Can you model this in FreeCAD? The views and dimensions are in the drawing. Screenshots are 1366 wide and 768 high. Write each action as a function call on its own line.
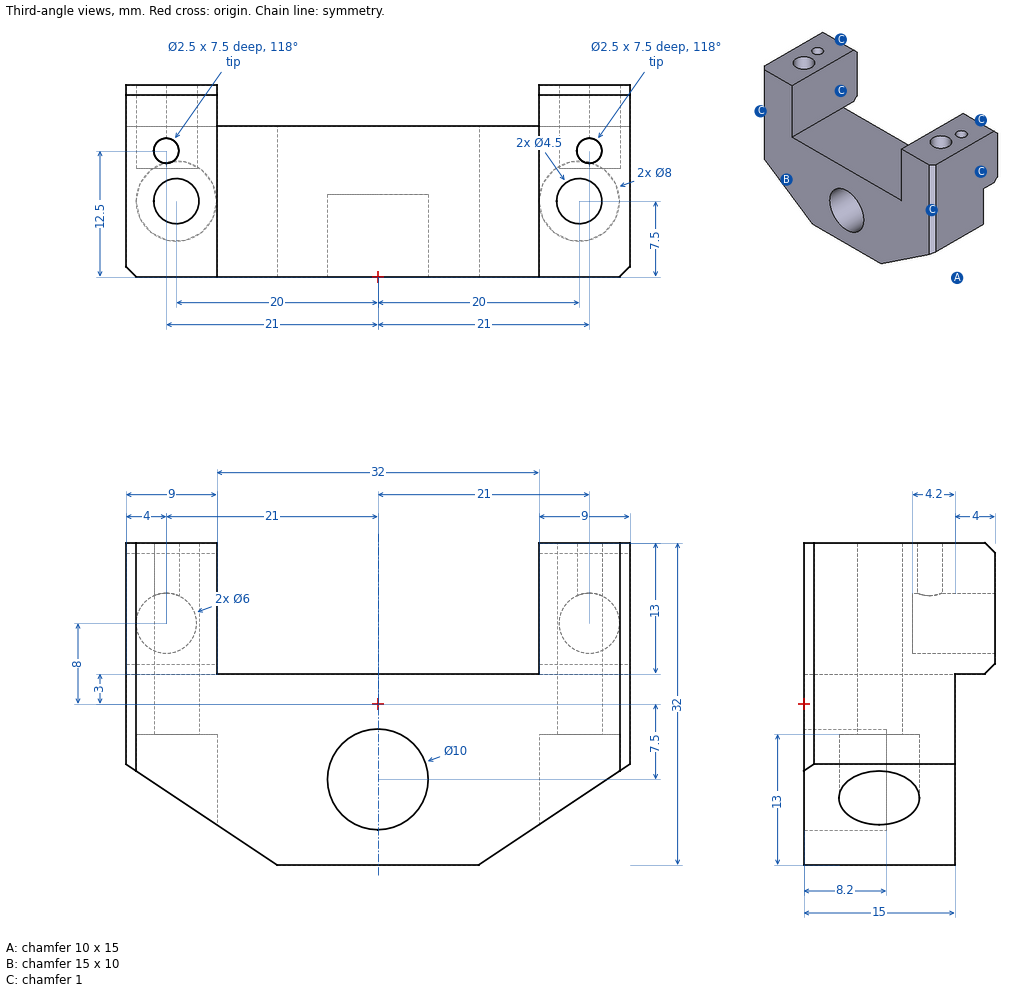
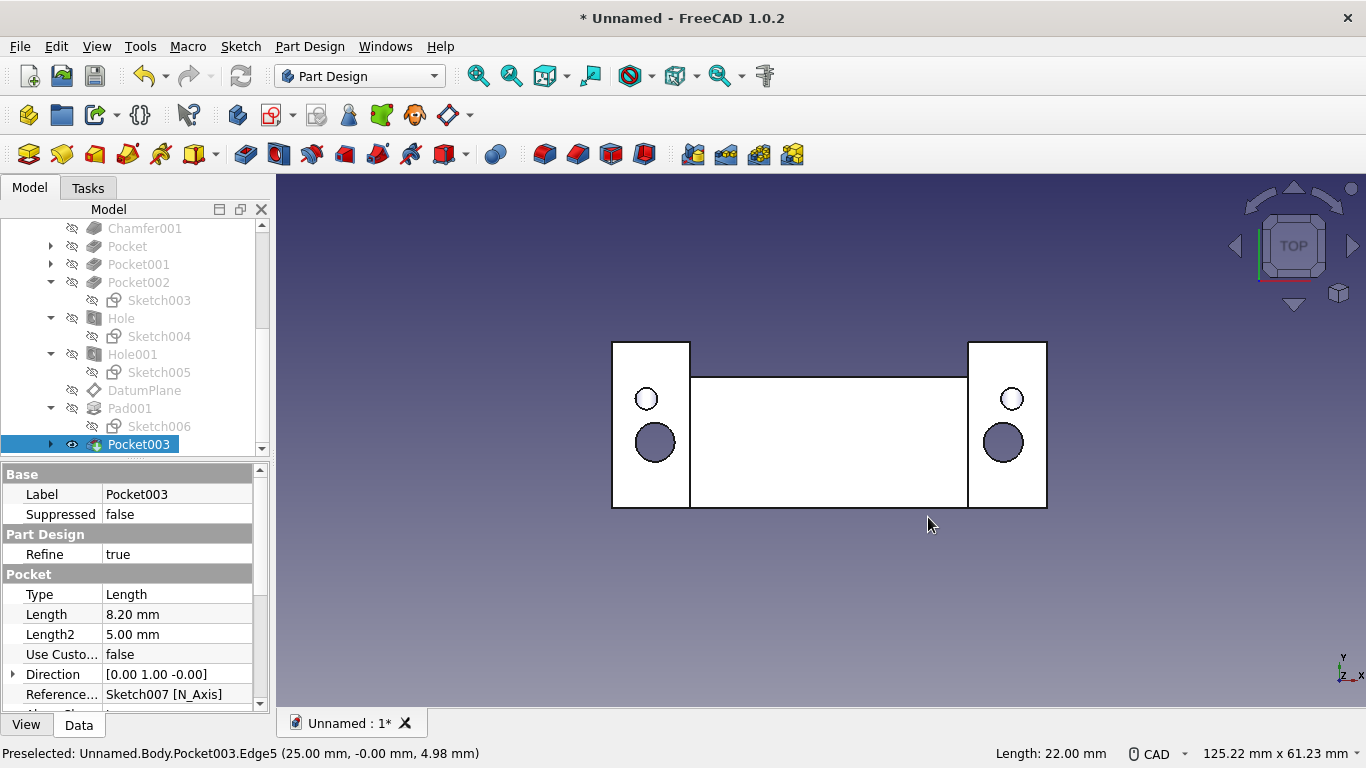
click(479, 76)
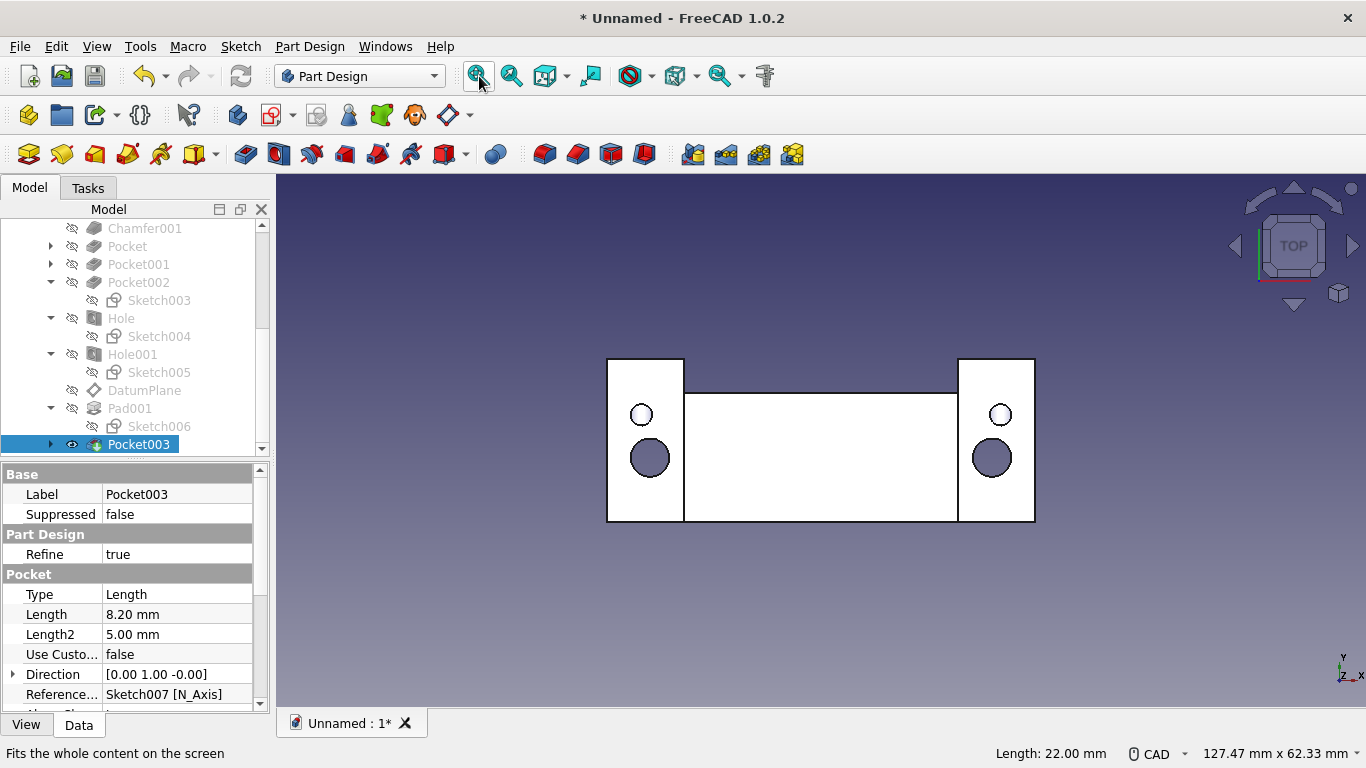
click(646, 358, ctrl)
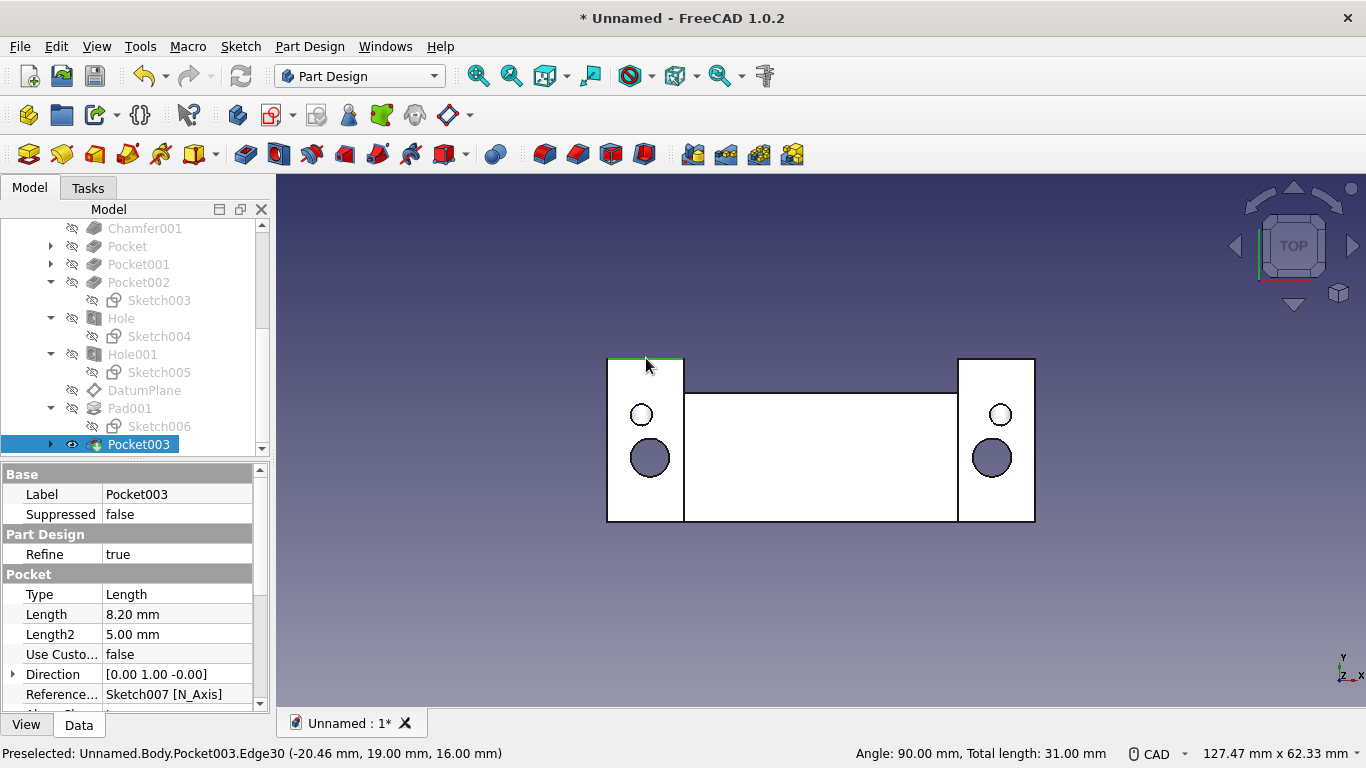
click(996, 358, ctrl)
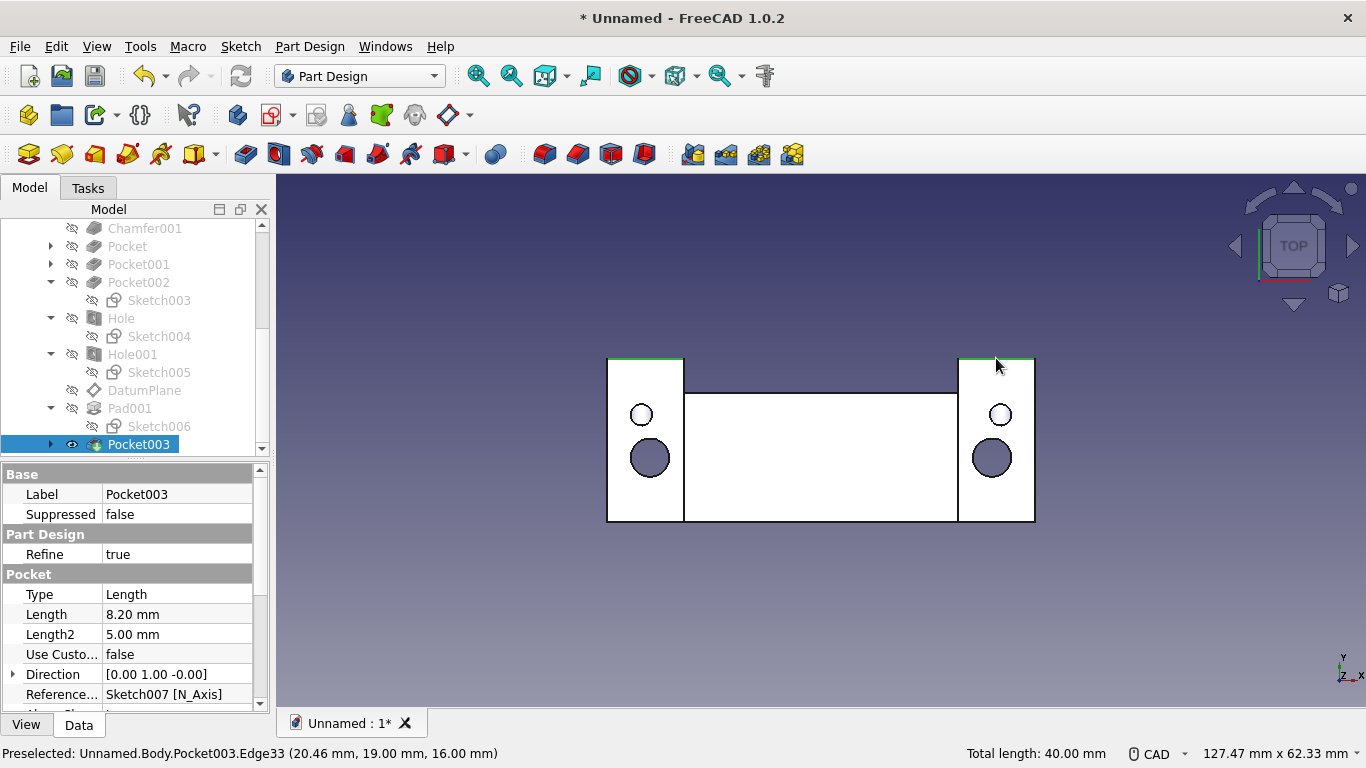
key(0)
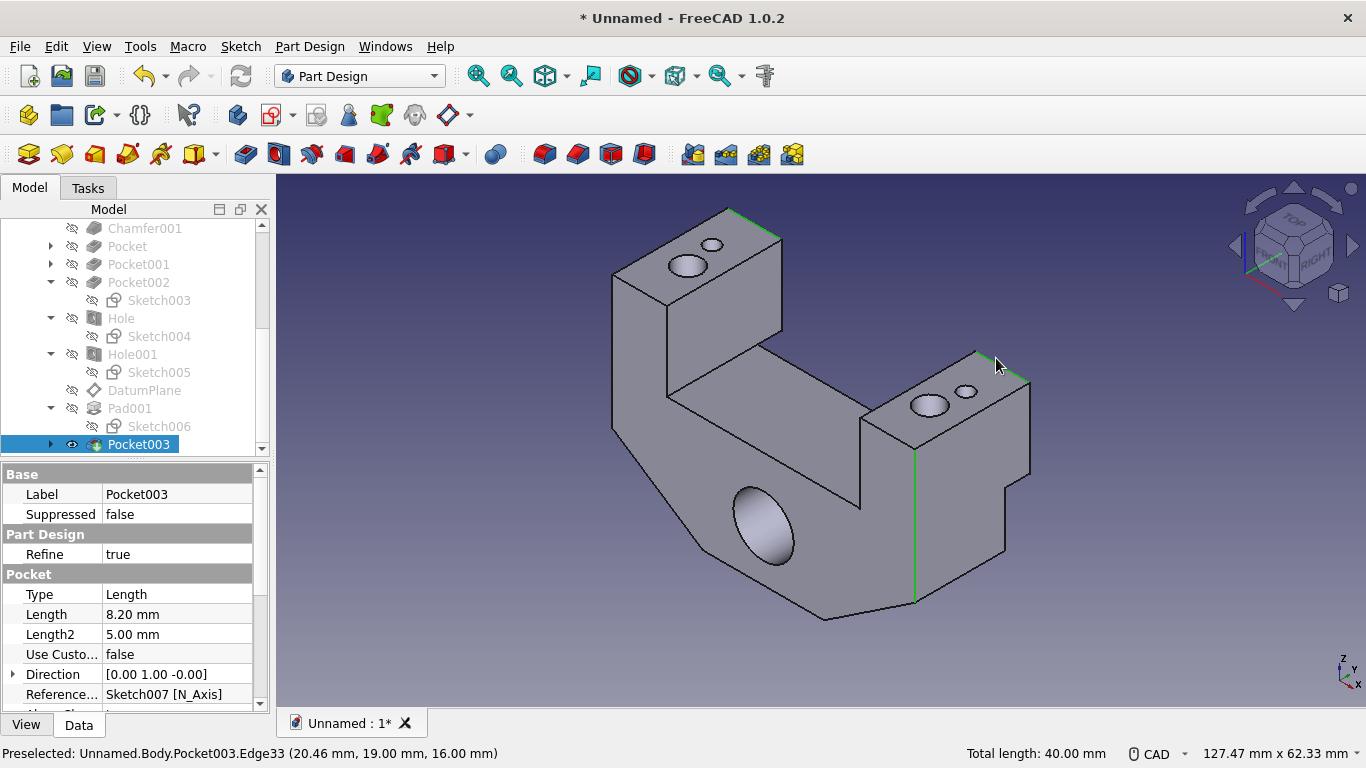
key(1)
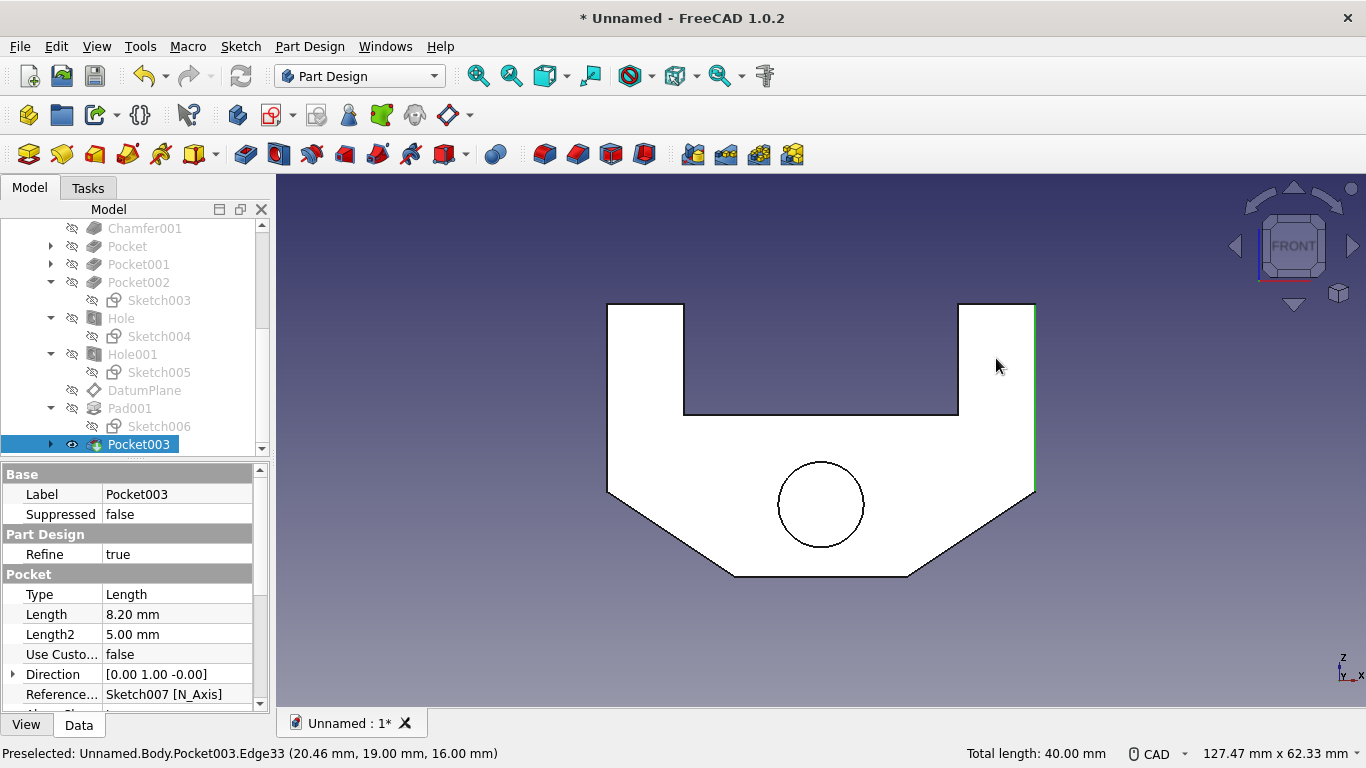
click(607, 434, ctrl)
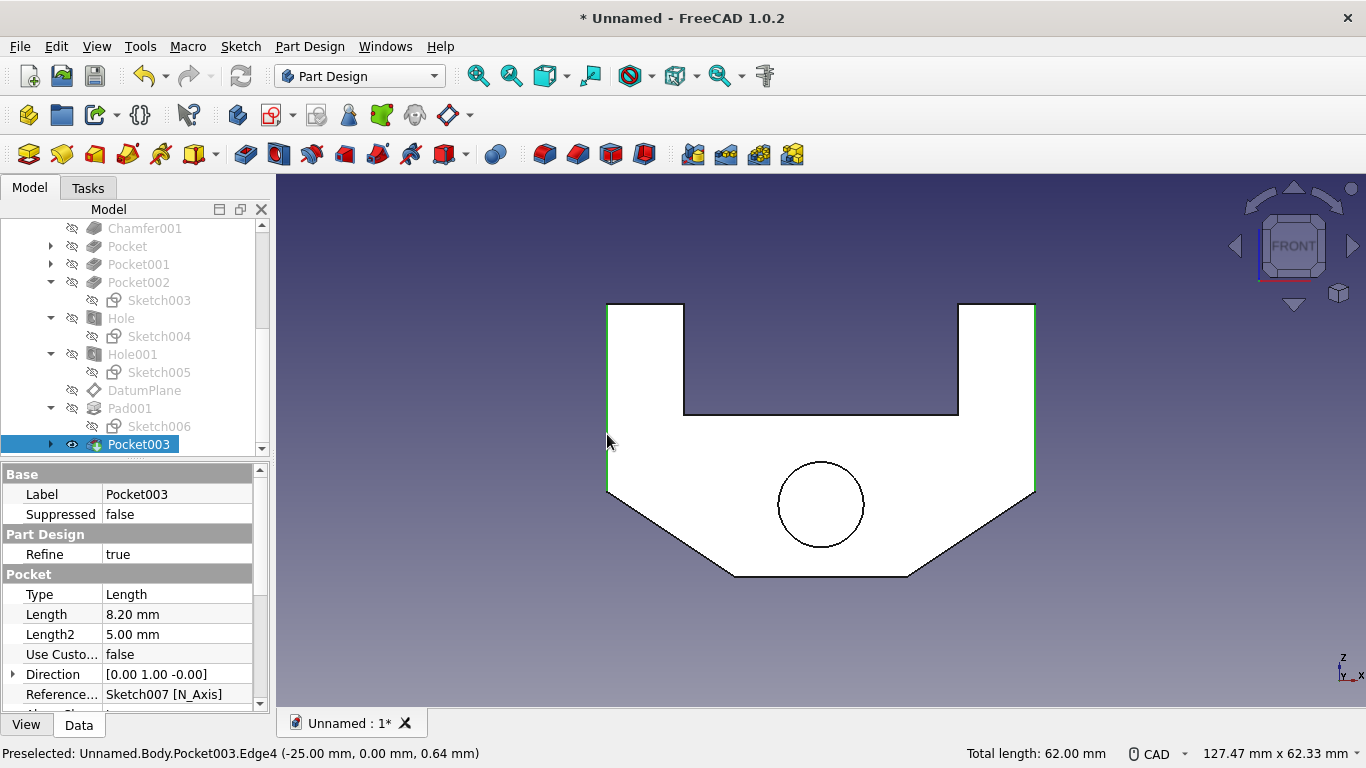
key(3)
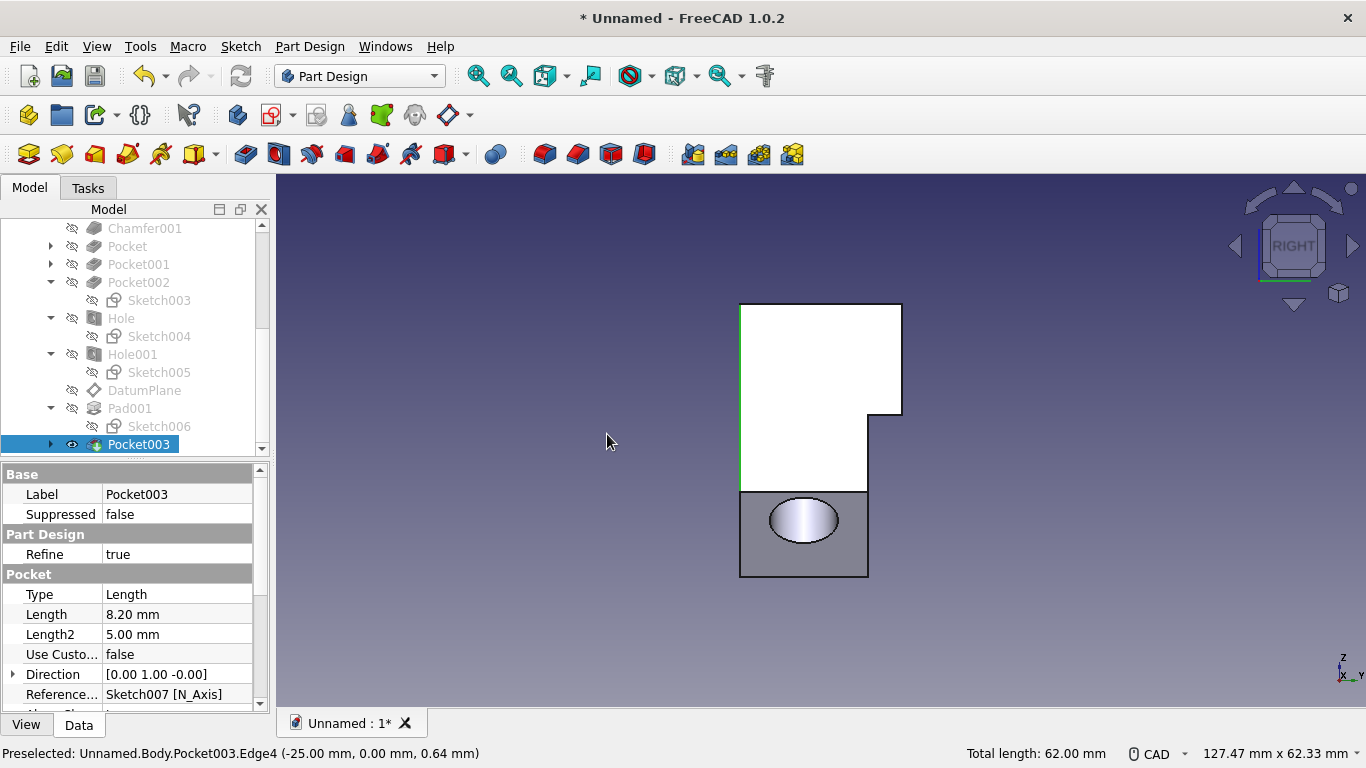
key(5)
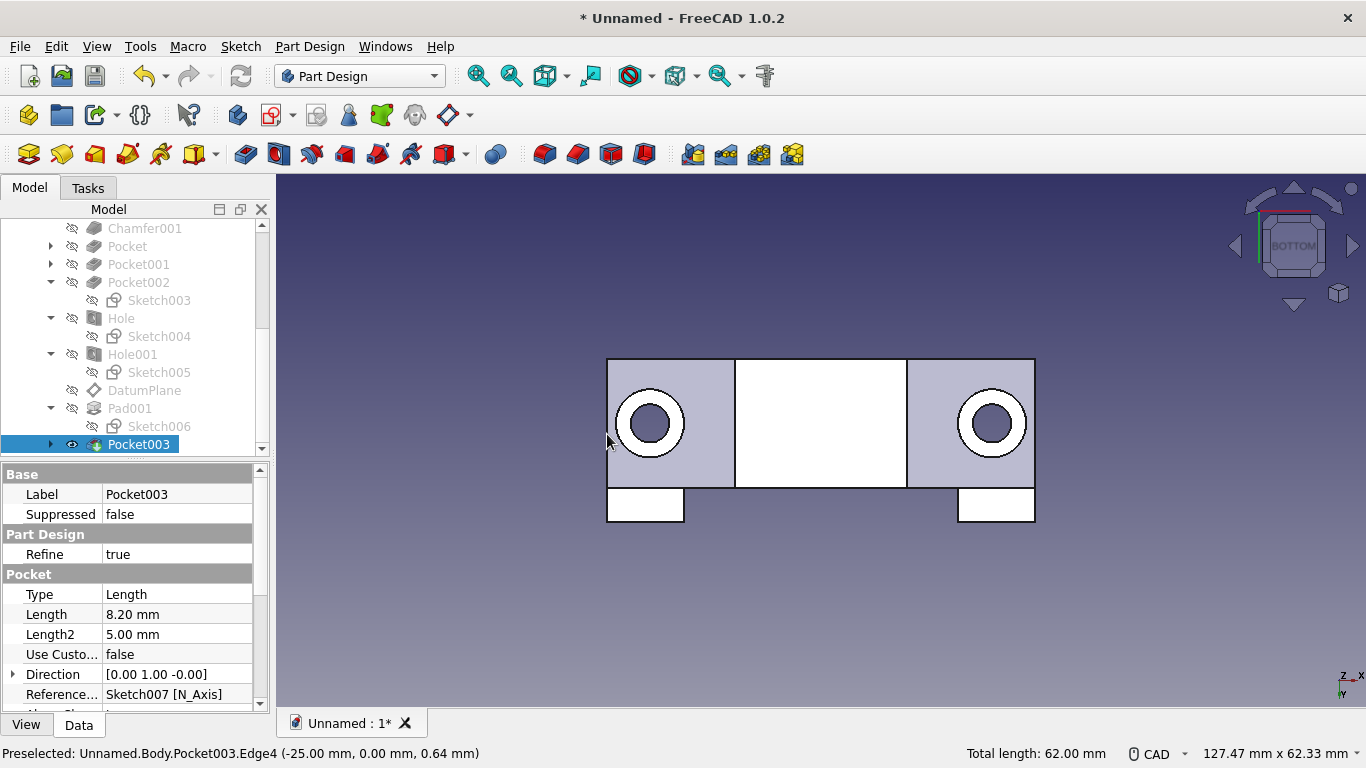
click(479, 76)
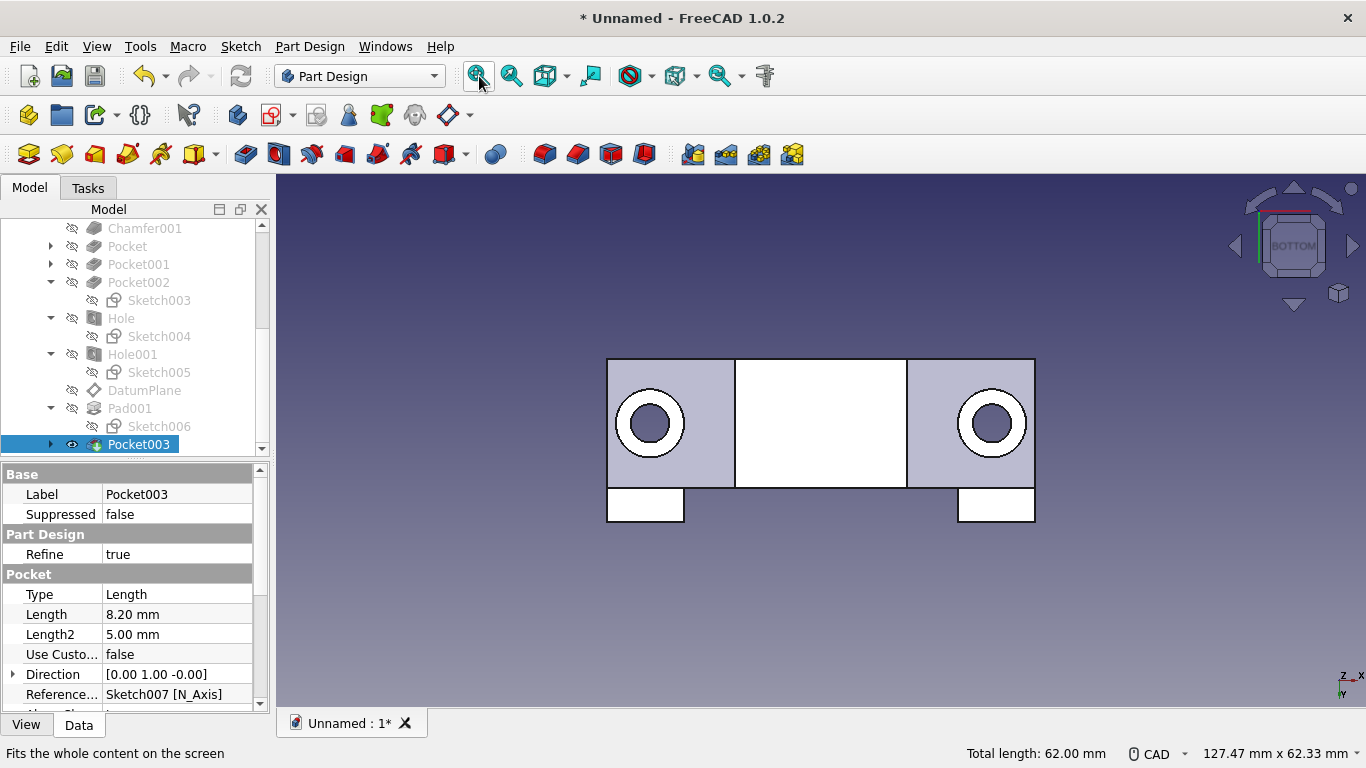
key(4)